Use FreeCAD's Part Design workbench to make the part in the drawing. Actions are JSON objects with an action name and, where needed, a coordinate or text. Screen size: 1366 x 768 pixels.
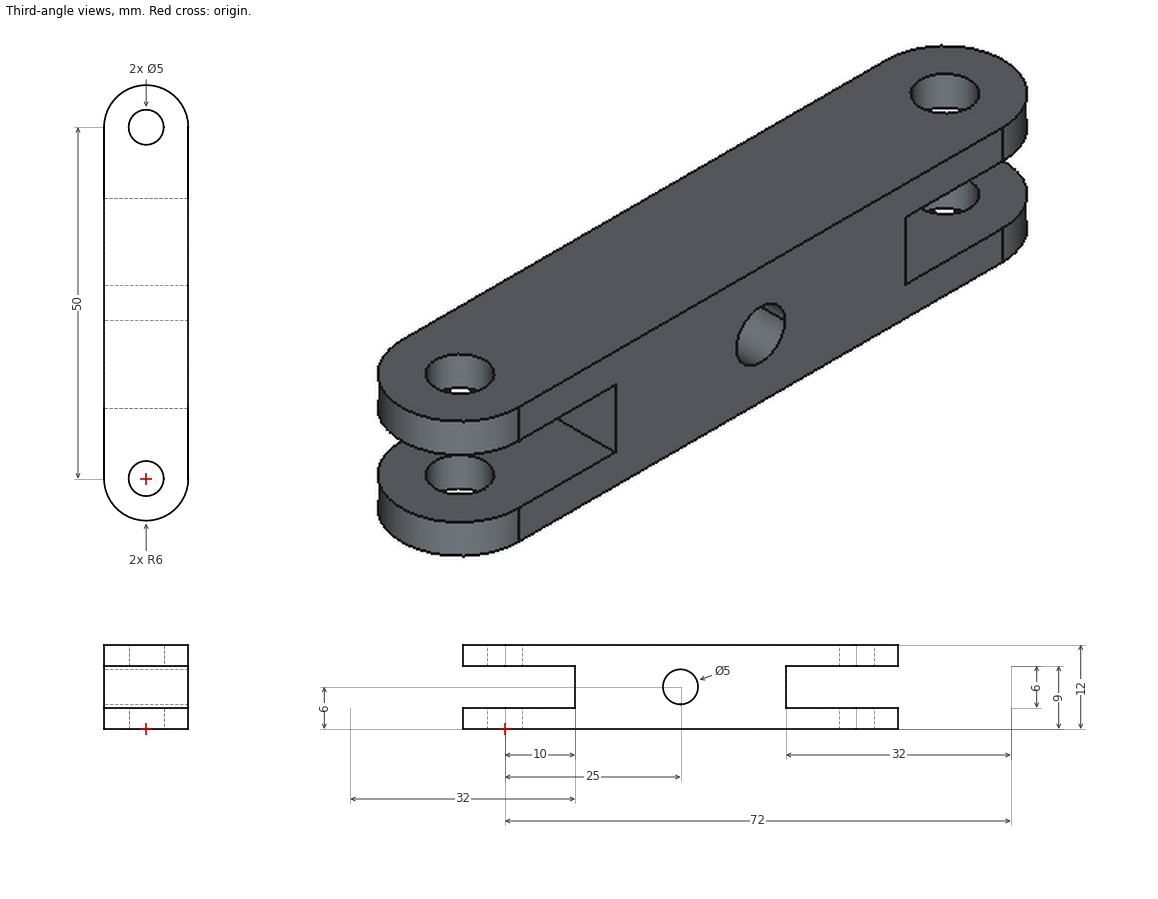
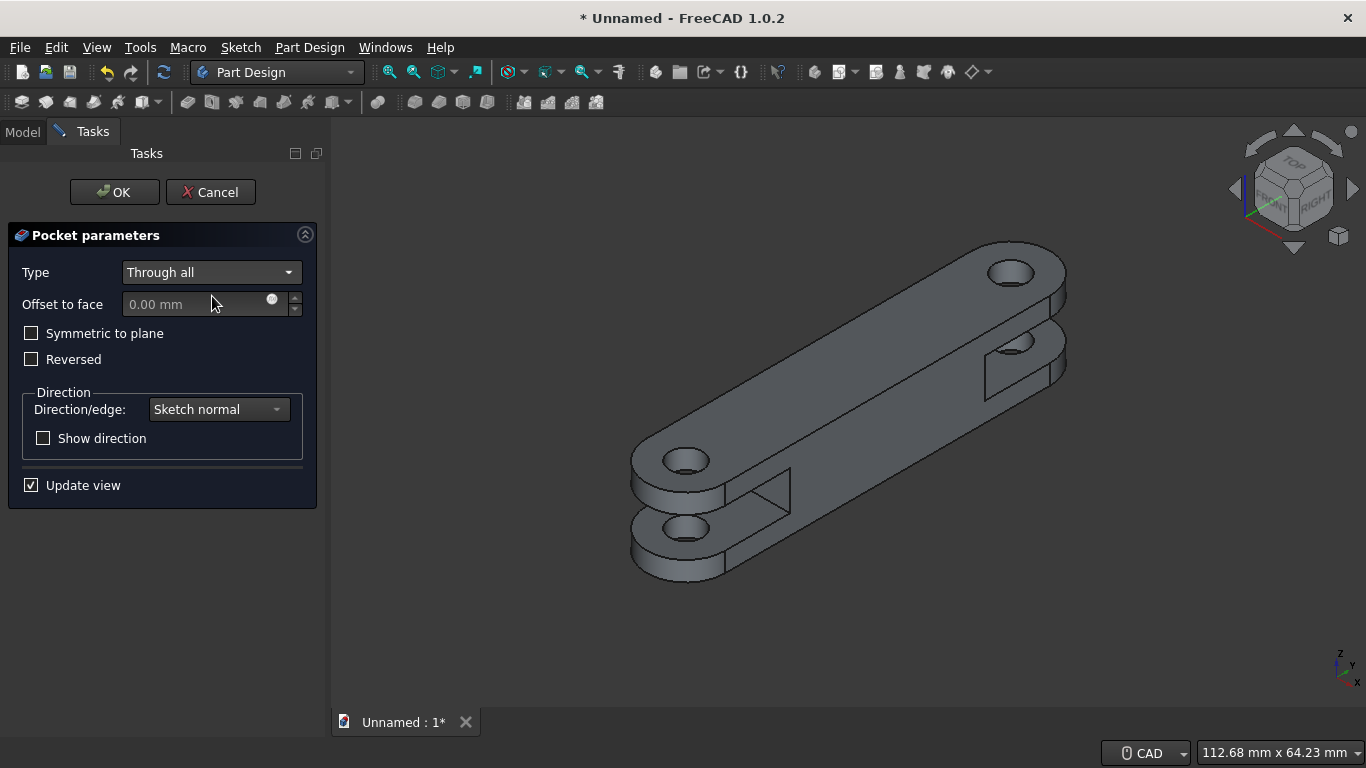
{"action": "left_click", "coordinate": [115, 192]}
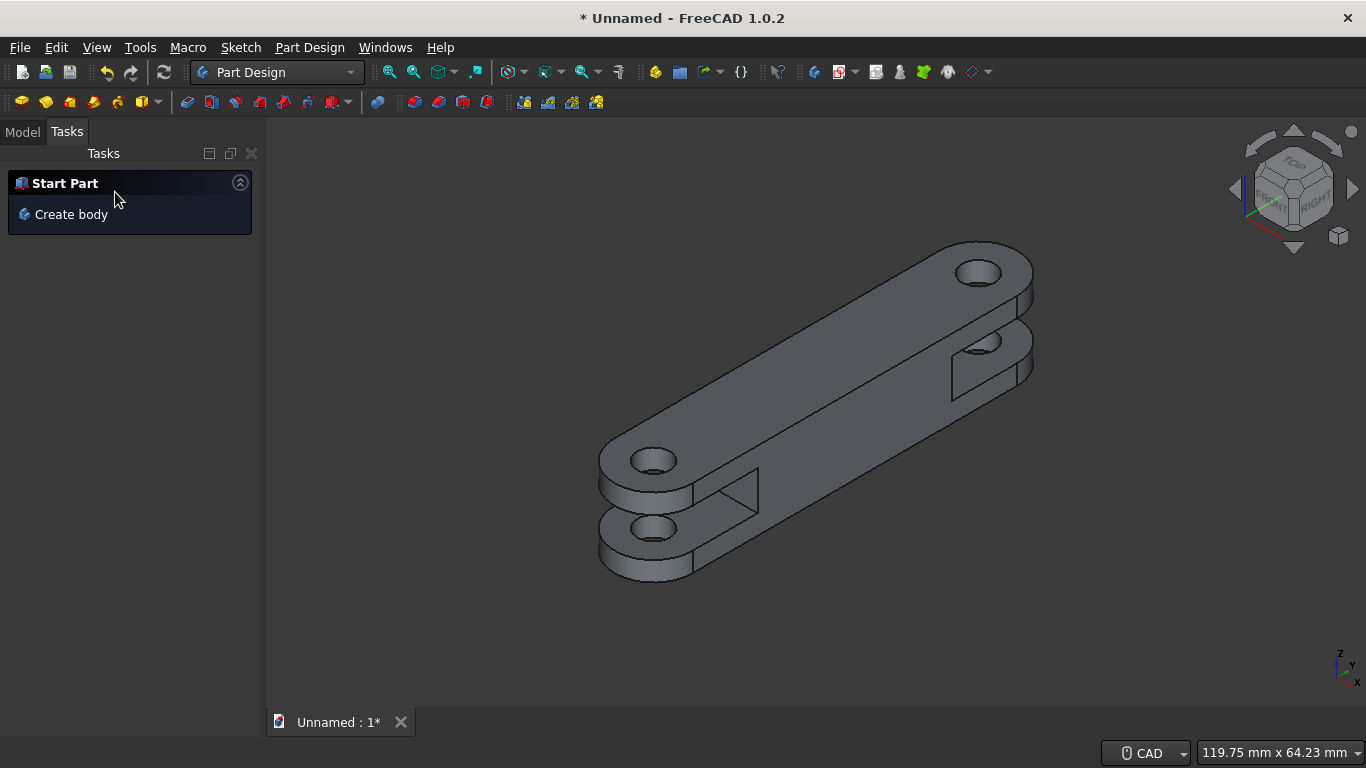
{"action": "left_click", "coordinate": [901, 407]}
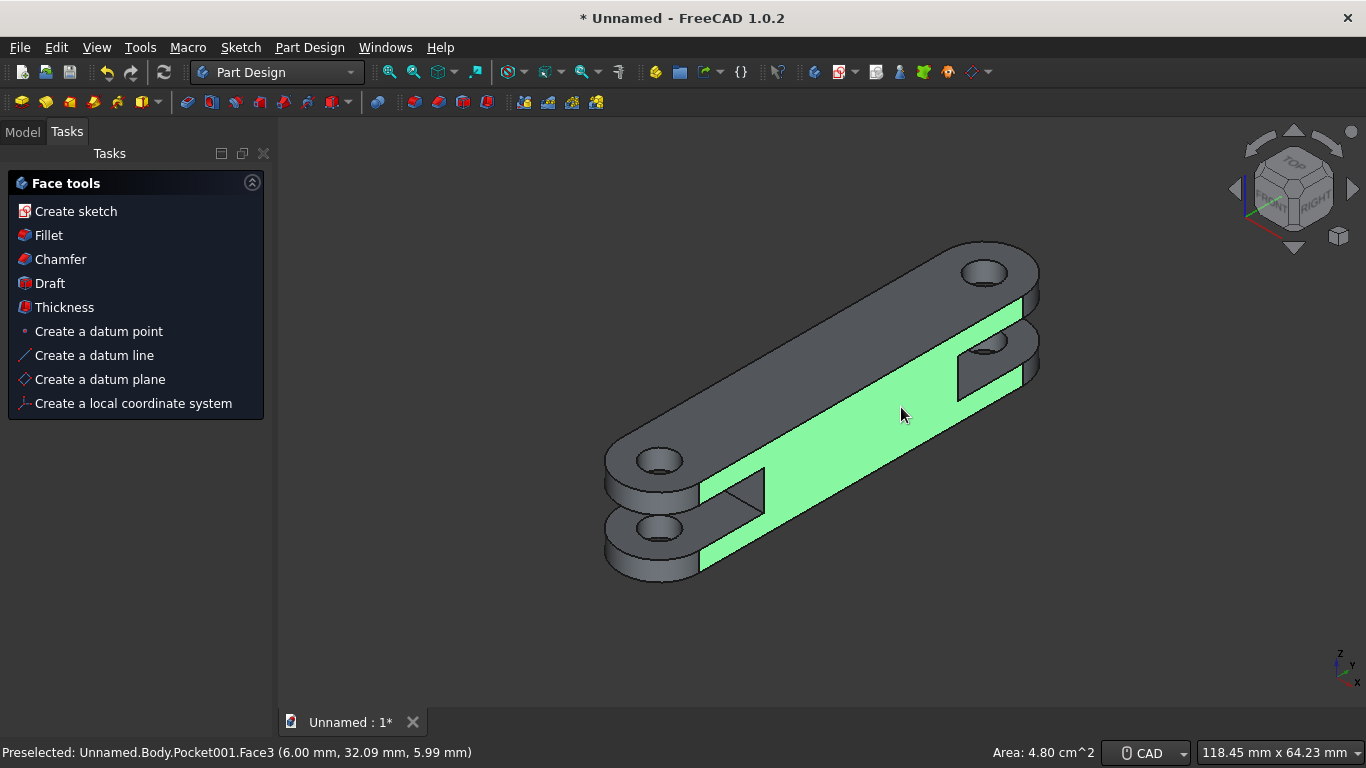
{"action": "left_click", "coordinate": [840, 72]}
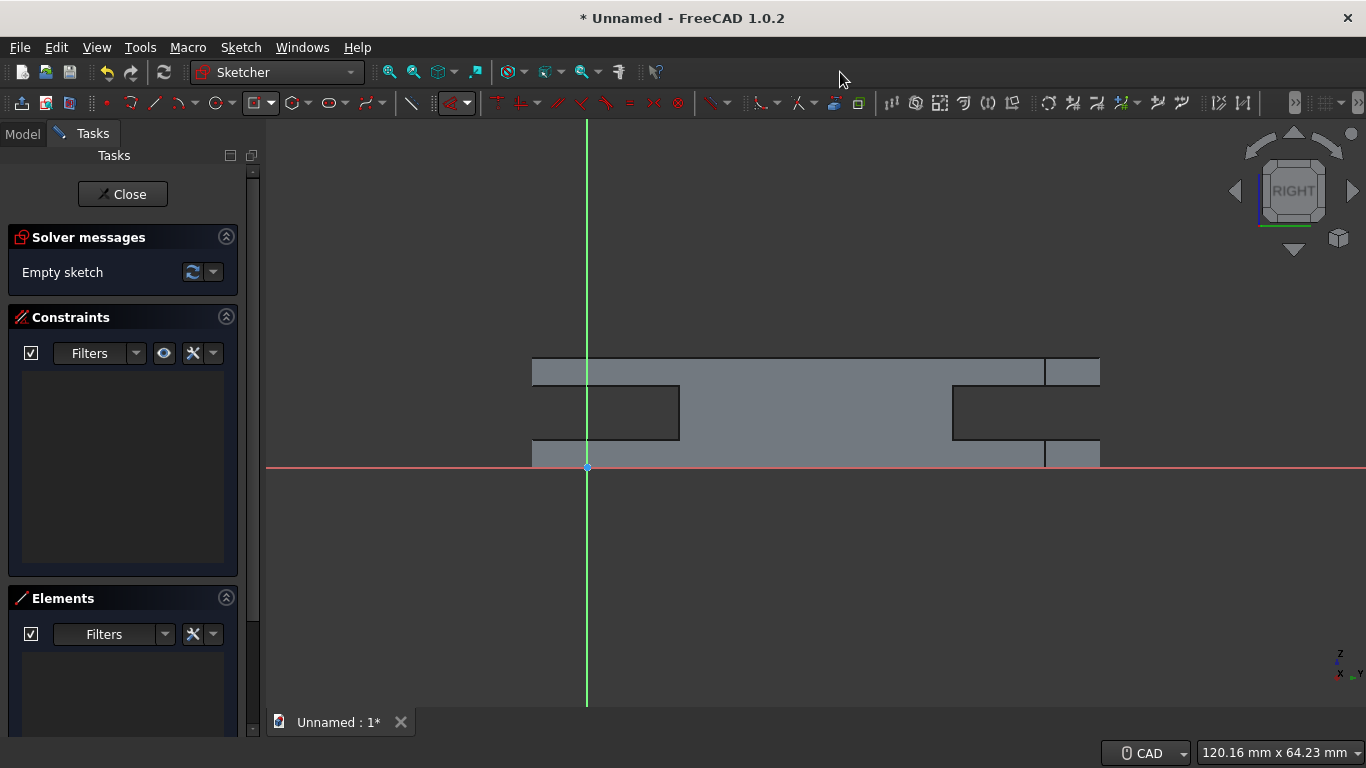
{"action": "scroll", "coordinate": [825, 413], "scroll_direction": "up", "scroll_amount": 11}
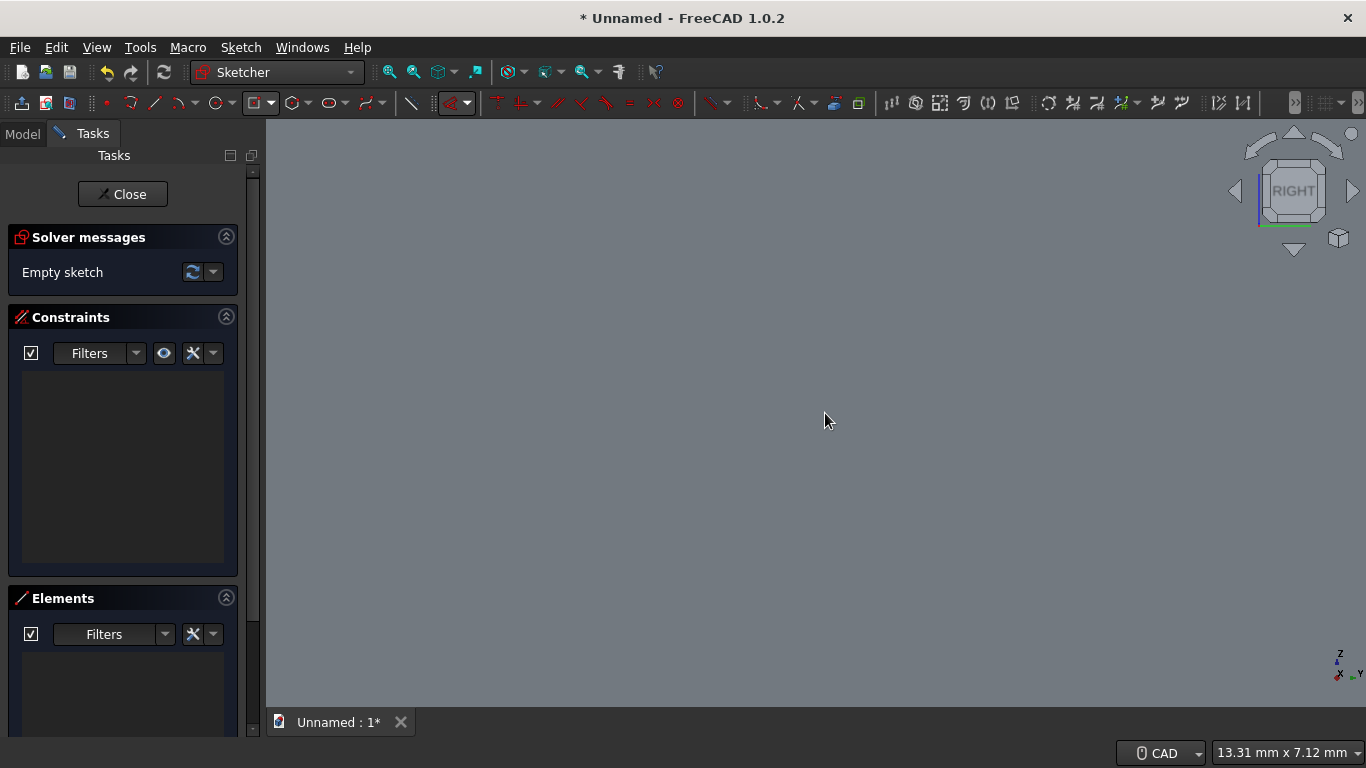
{"action": "left_click", "coordinate": [216, 104]}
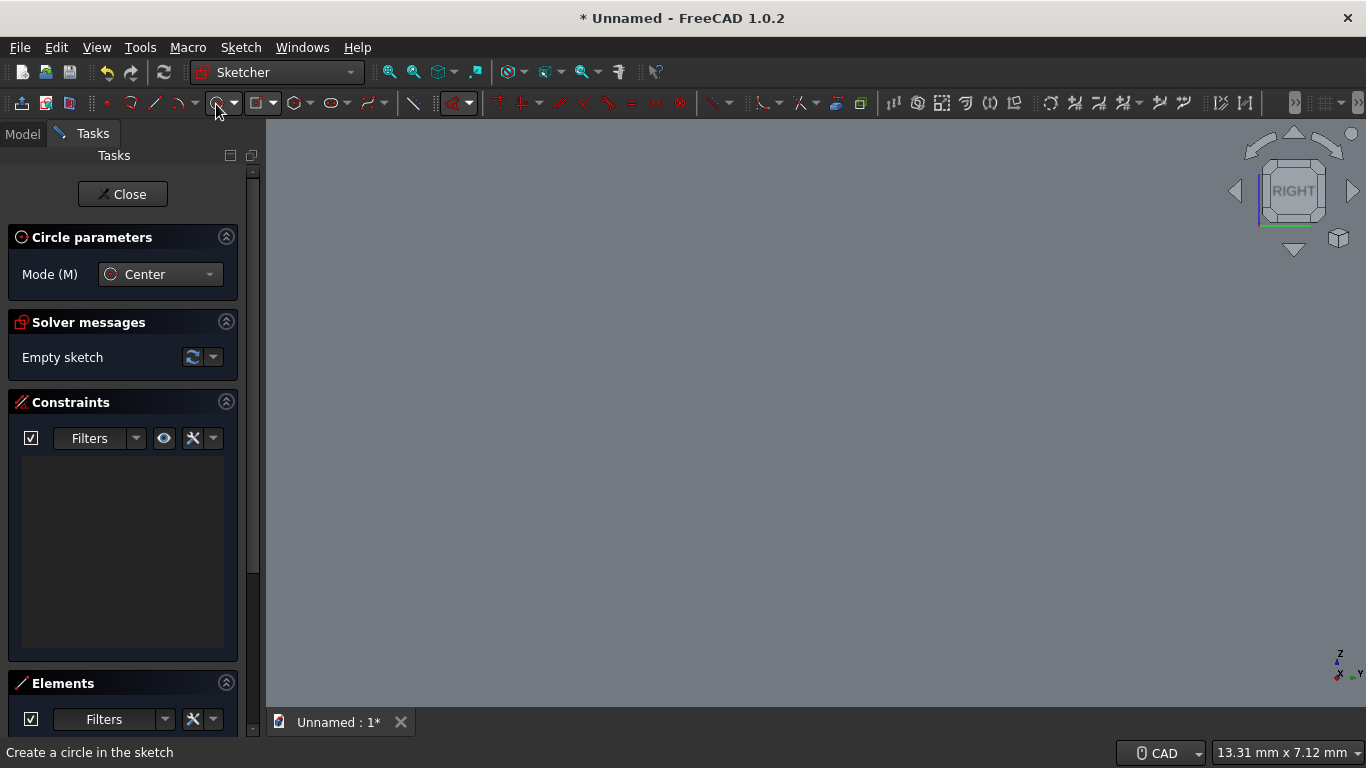
{"action": "left_click", "coordinate": [740, 409]}
{"action": "left_click", "coordinate": [886, 263]}
{"action": "key", "text": "Escape"}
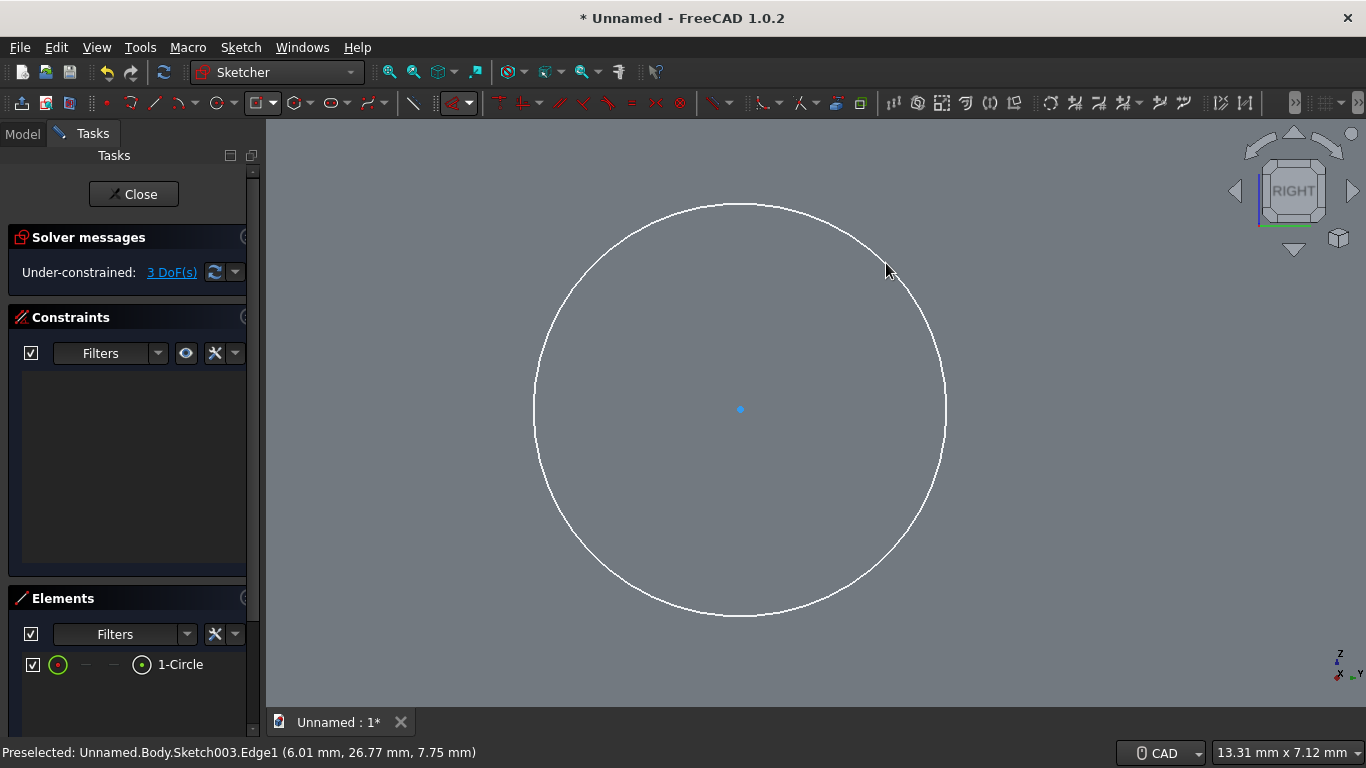
{"action": "left_click", "coordinate": [886, 264]}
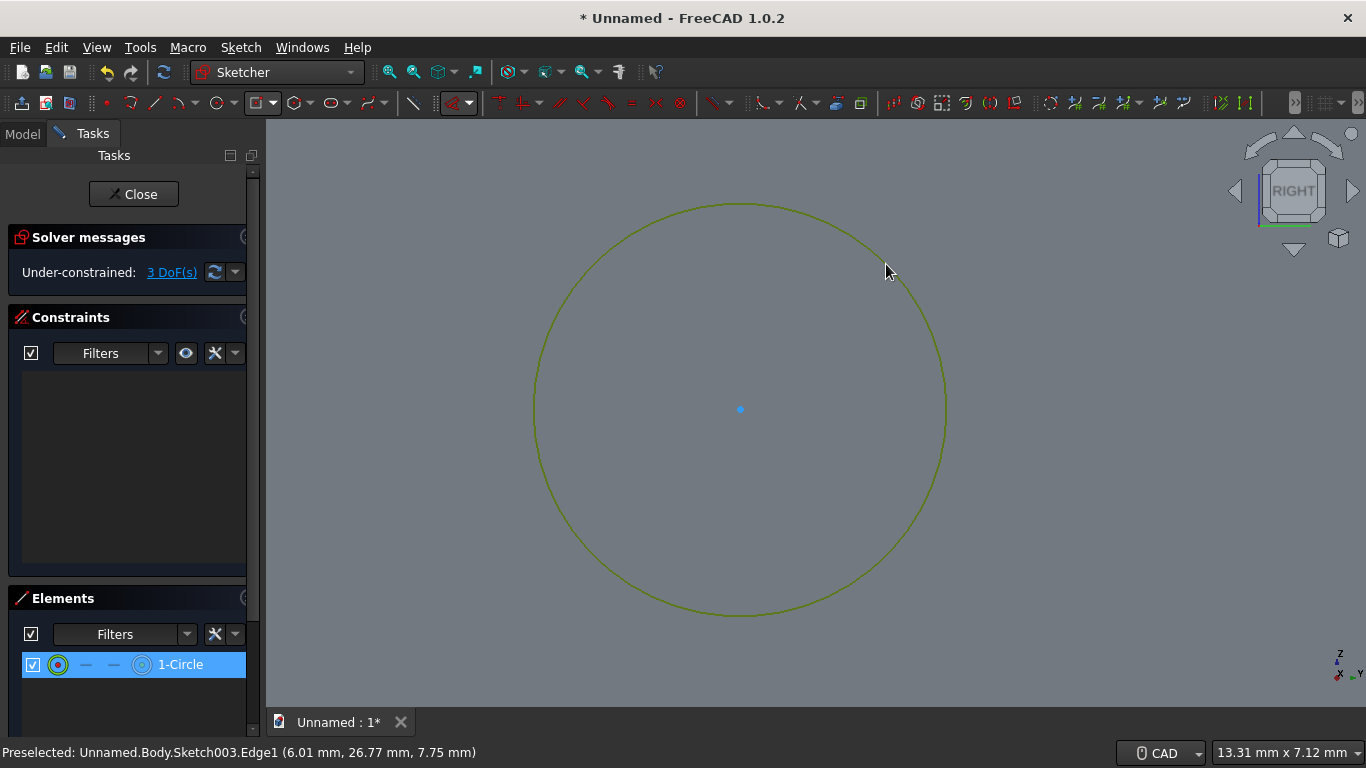
{"action": "key", "text": "k o"}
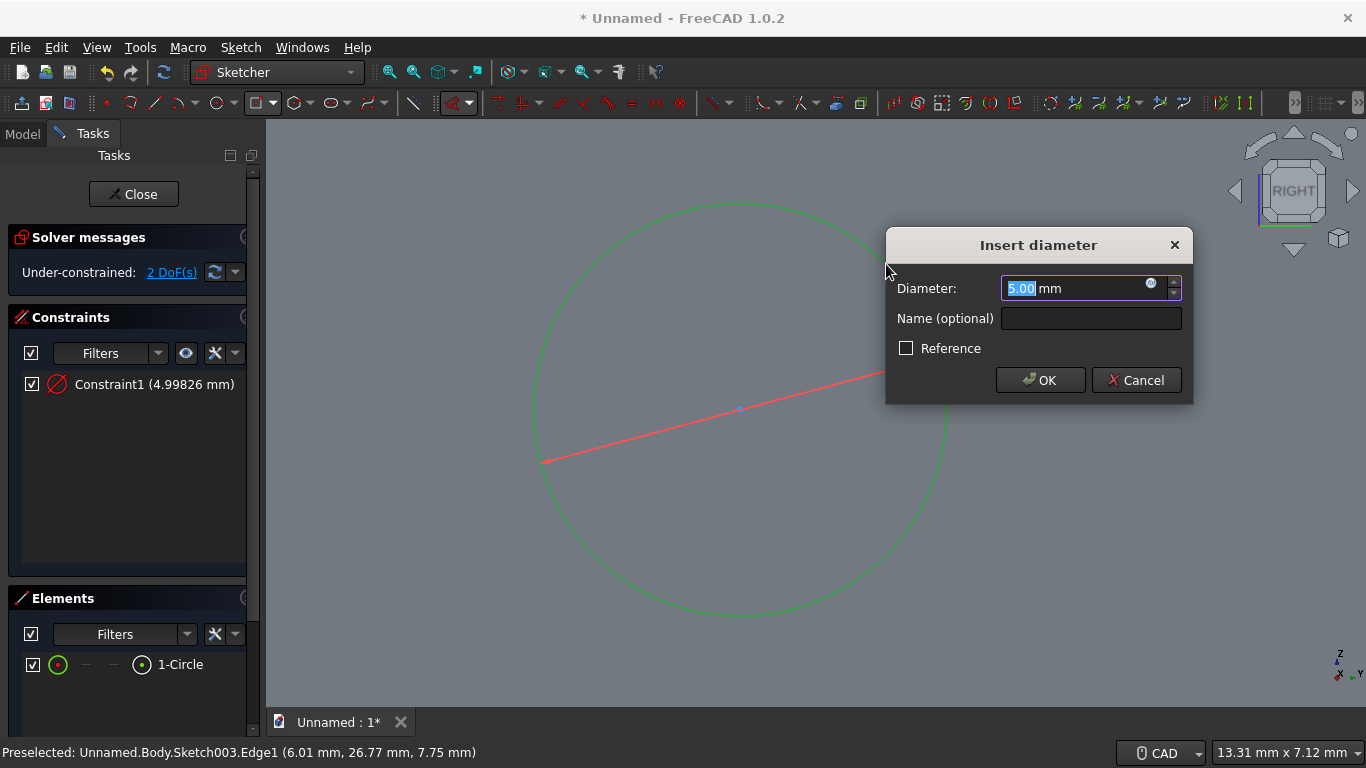
{"action": "type", "text": "5"}
{"action": "key", "text": "Return"}